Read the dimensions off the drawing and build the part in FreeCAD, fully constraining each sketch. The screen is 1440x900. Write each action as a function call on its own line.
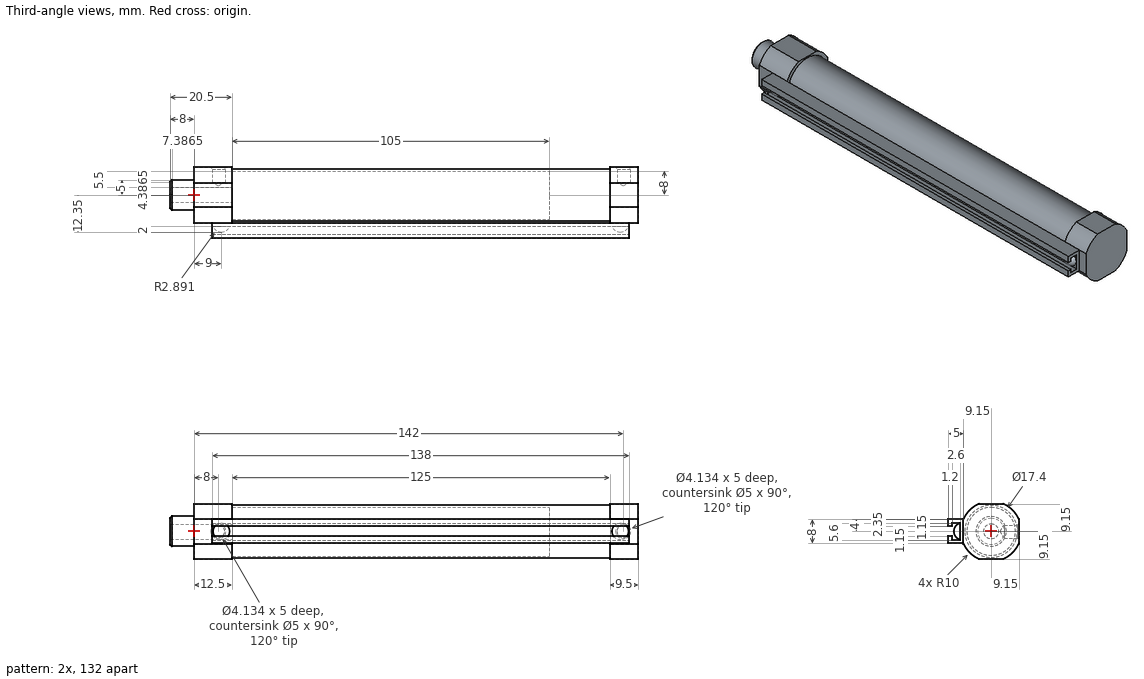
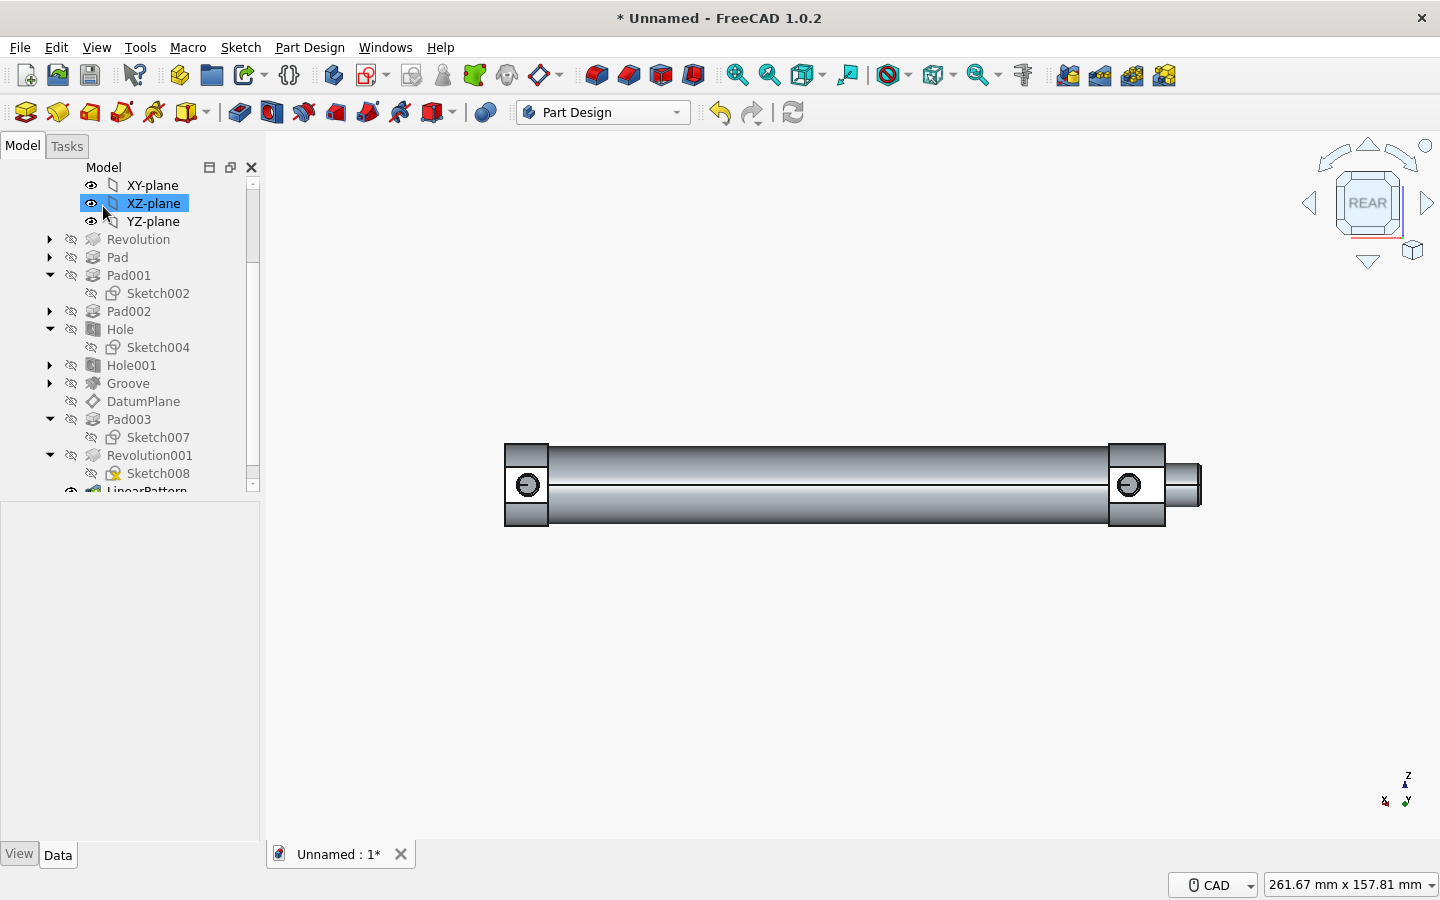
key(0)